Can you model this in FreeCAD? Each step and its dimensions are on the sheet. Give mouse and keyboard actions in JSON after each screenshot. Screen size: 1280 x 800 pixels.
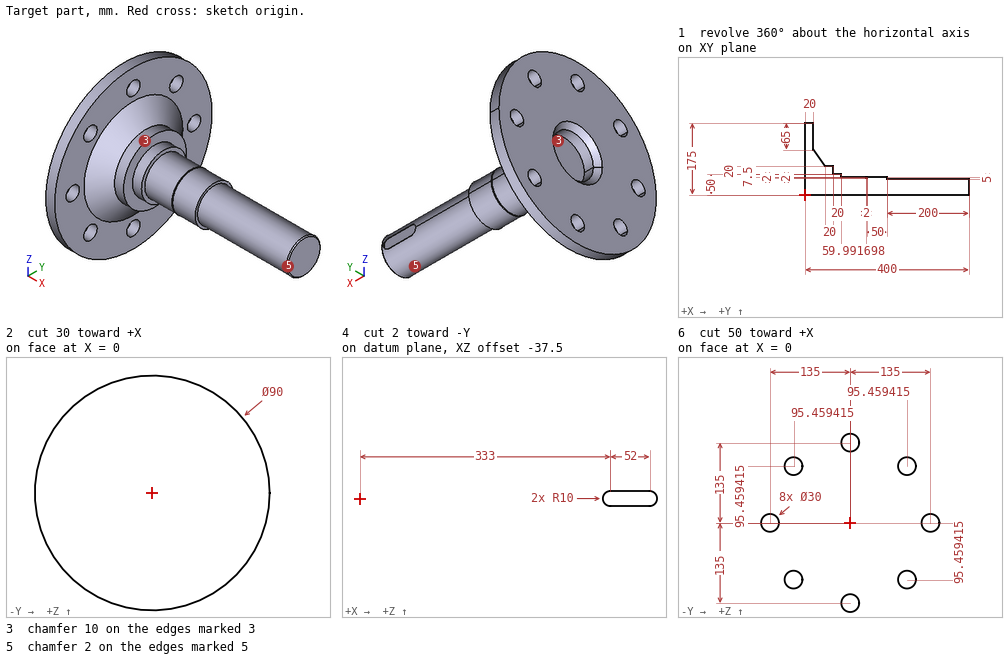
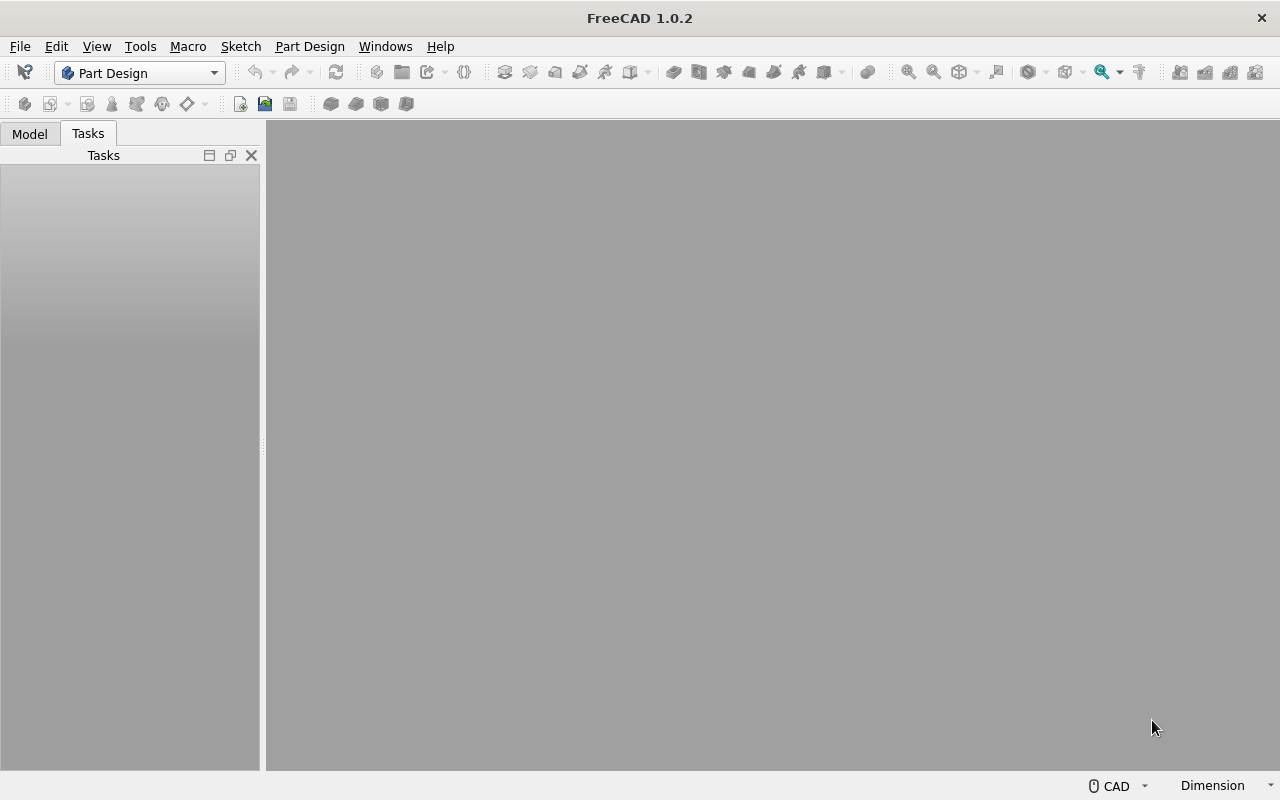
{"action": "left_click", "coordinate": [240, 104]}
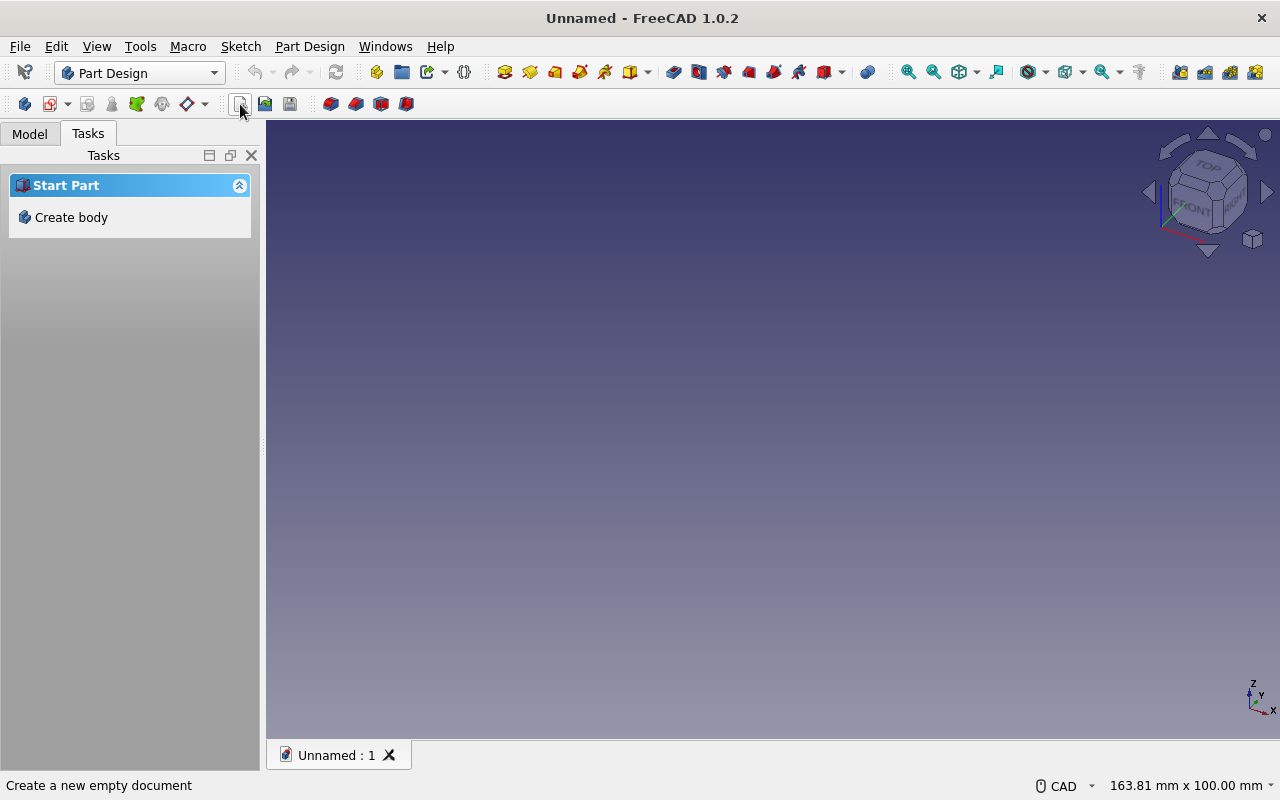
{"action": "left_click", "coordinate": [50, 104]}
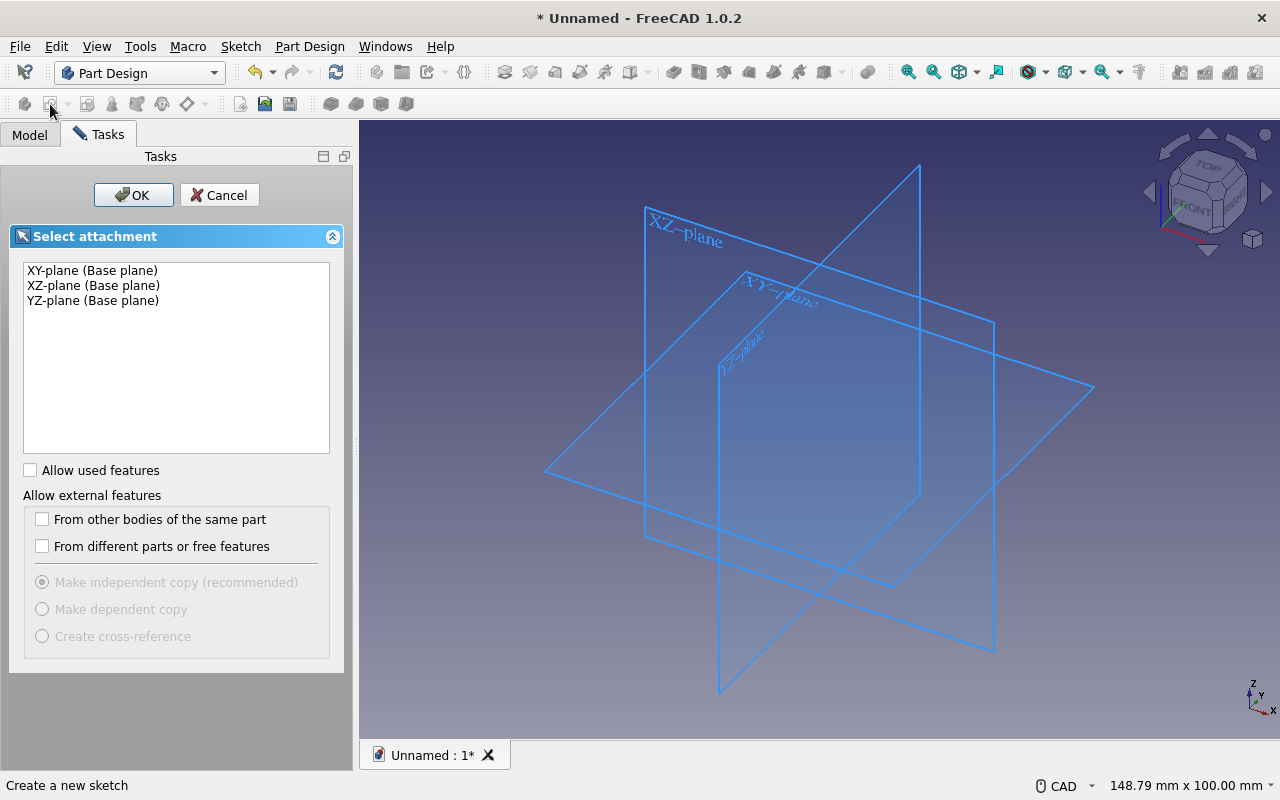
{"action": "left_click", "coordinate": [84, 270]}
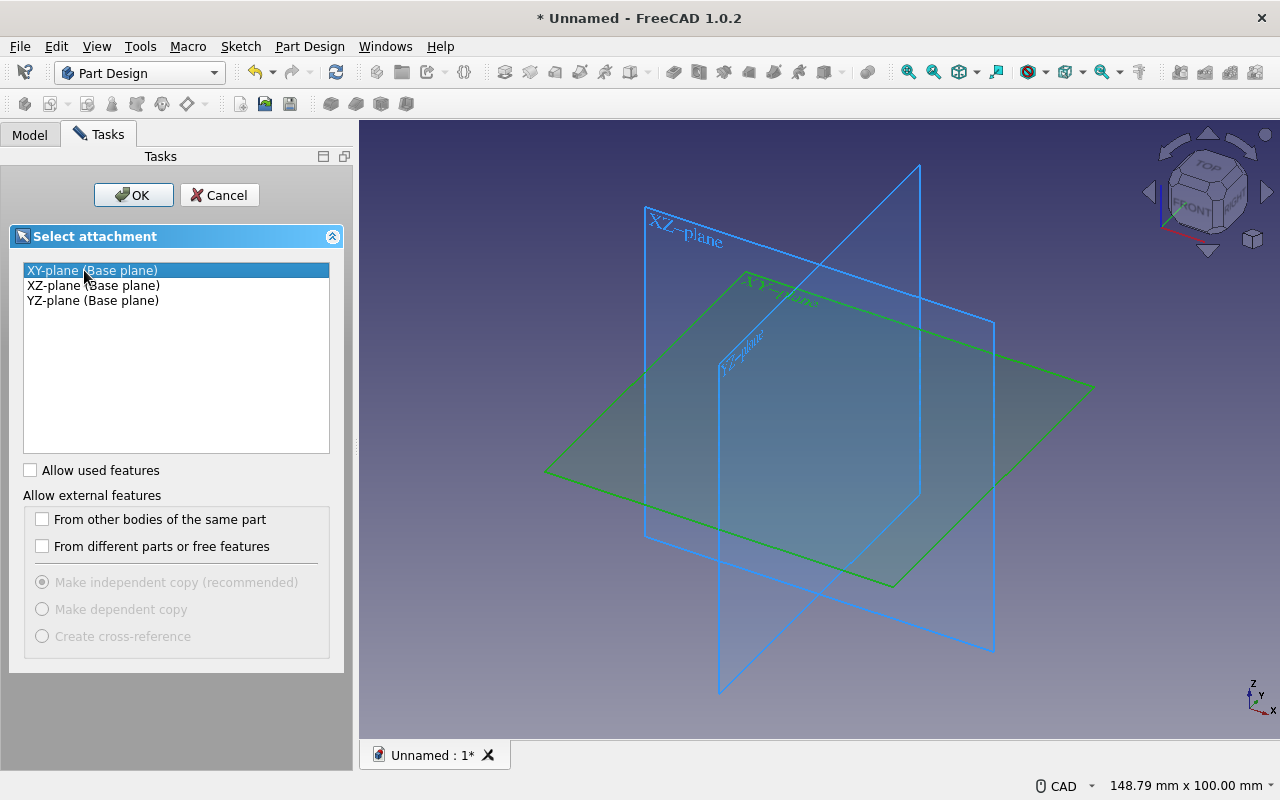
{"action": "left_click", "coordinate": [134, 195]}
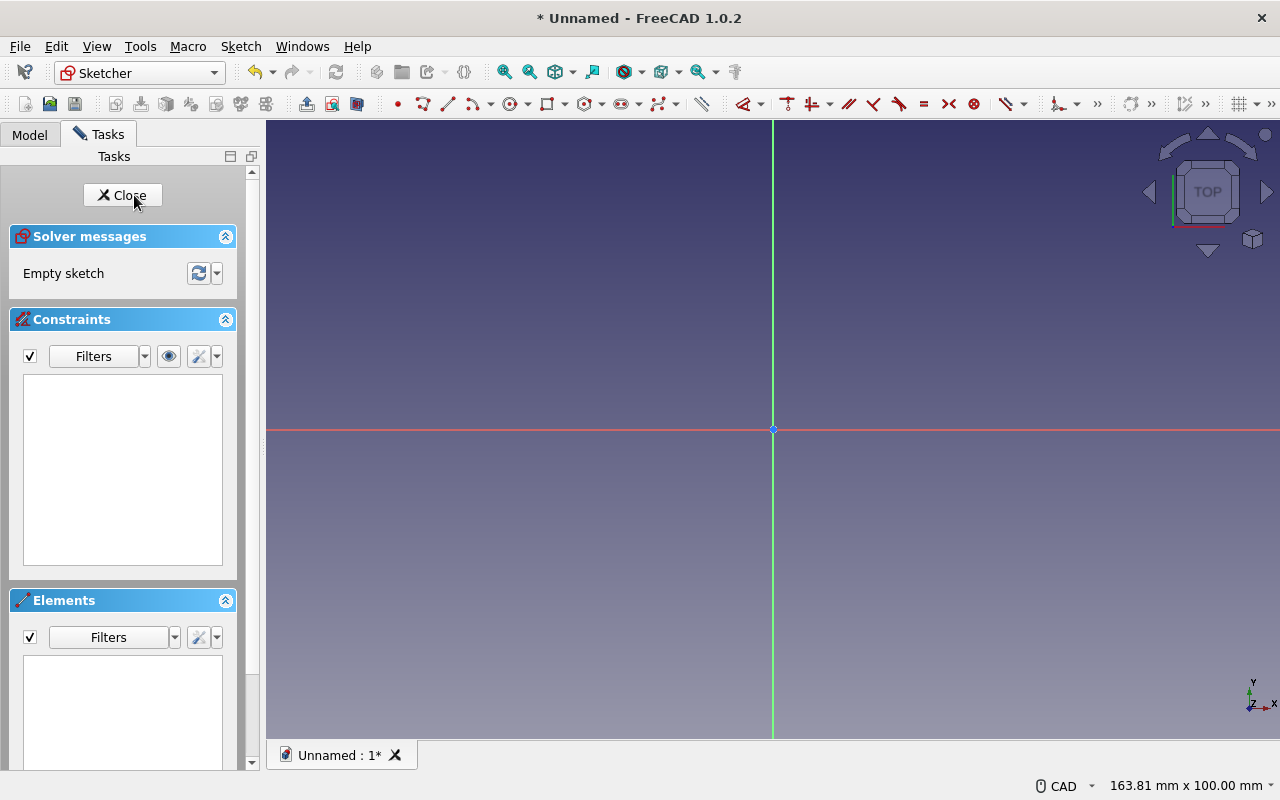
{"action": "scroll", "coordinate": [294, 607], "scroll_direction": "down", "scroll_amount": 7}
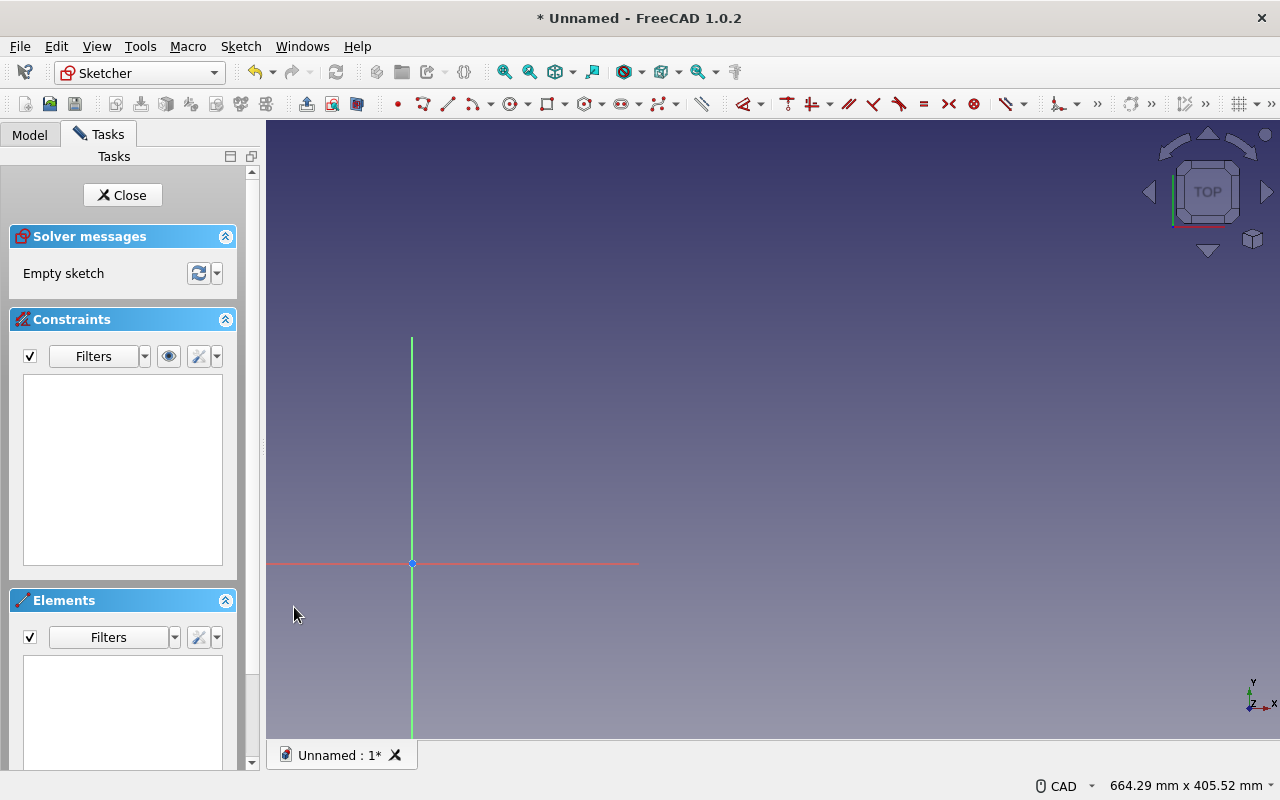
{"action": "left_click", "coordinate": [423, 104]}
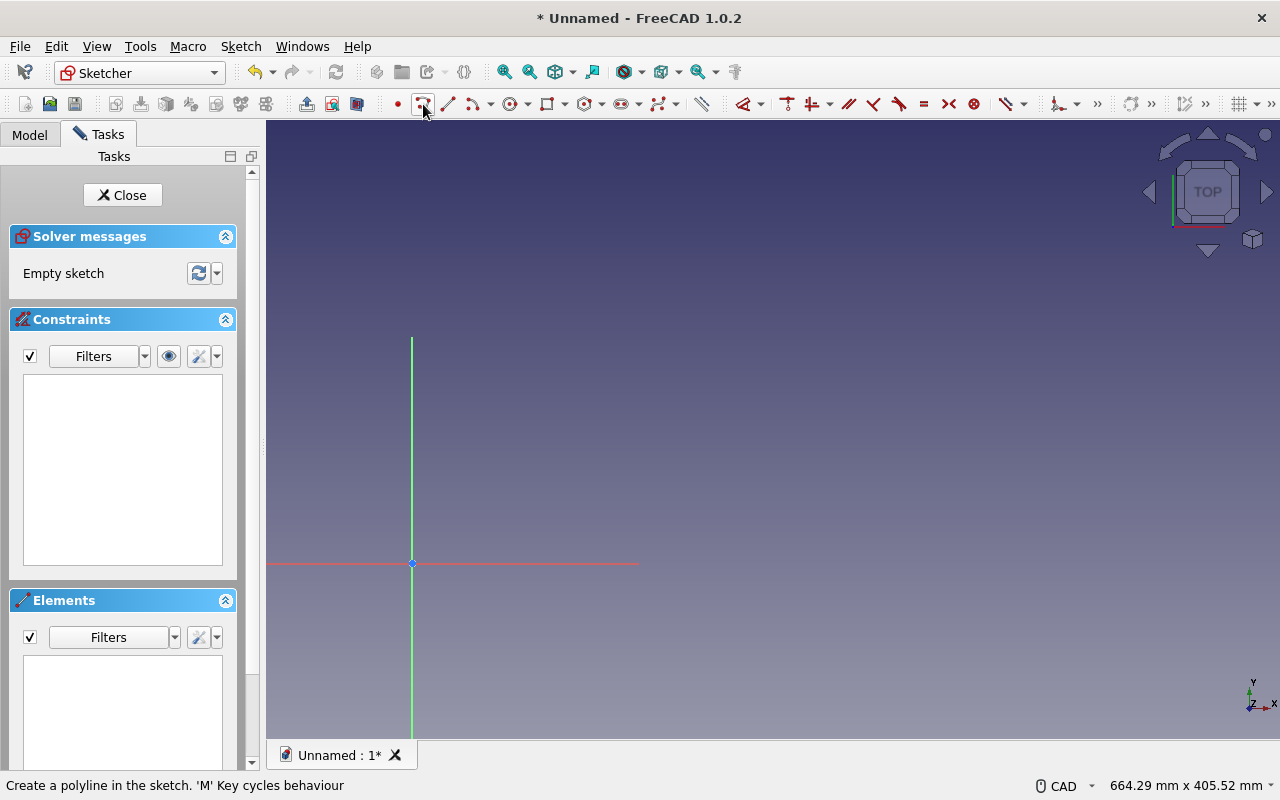
{"action": "left_click", "coordinate": [412, 564]}
{"action": "left_click", "coordinate": [1023, 555]}
{"action": "left_click", "coordinate": [1023, 507]}
{"action": "left_click", "coordinate": [717, 507]}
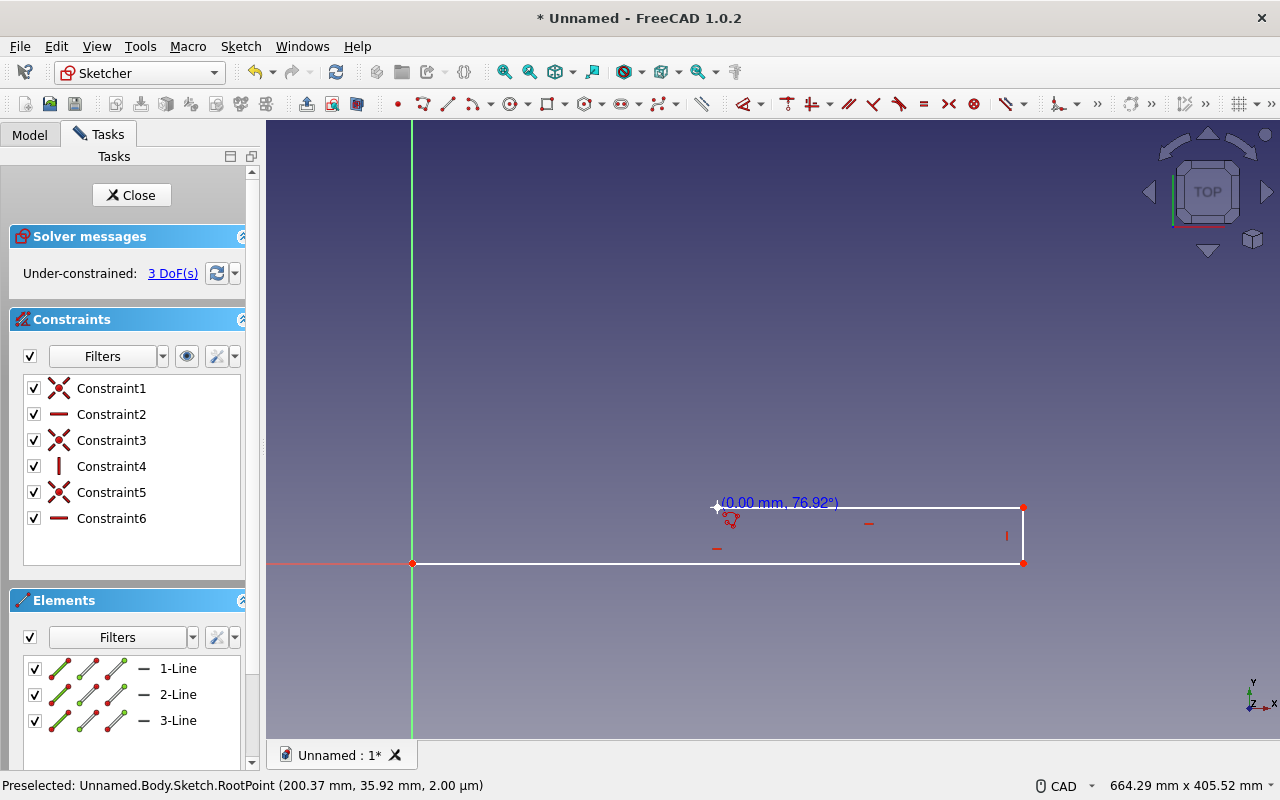
{"action": "scroll", "coordinate": [717, 499], "scroll_direction": "up", "scroll_amount": 4}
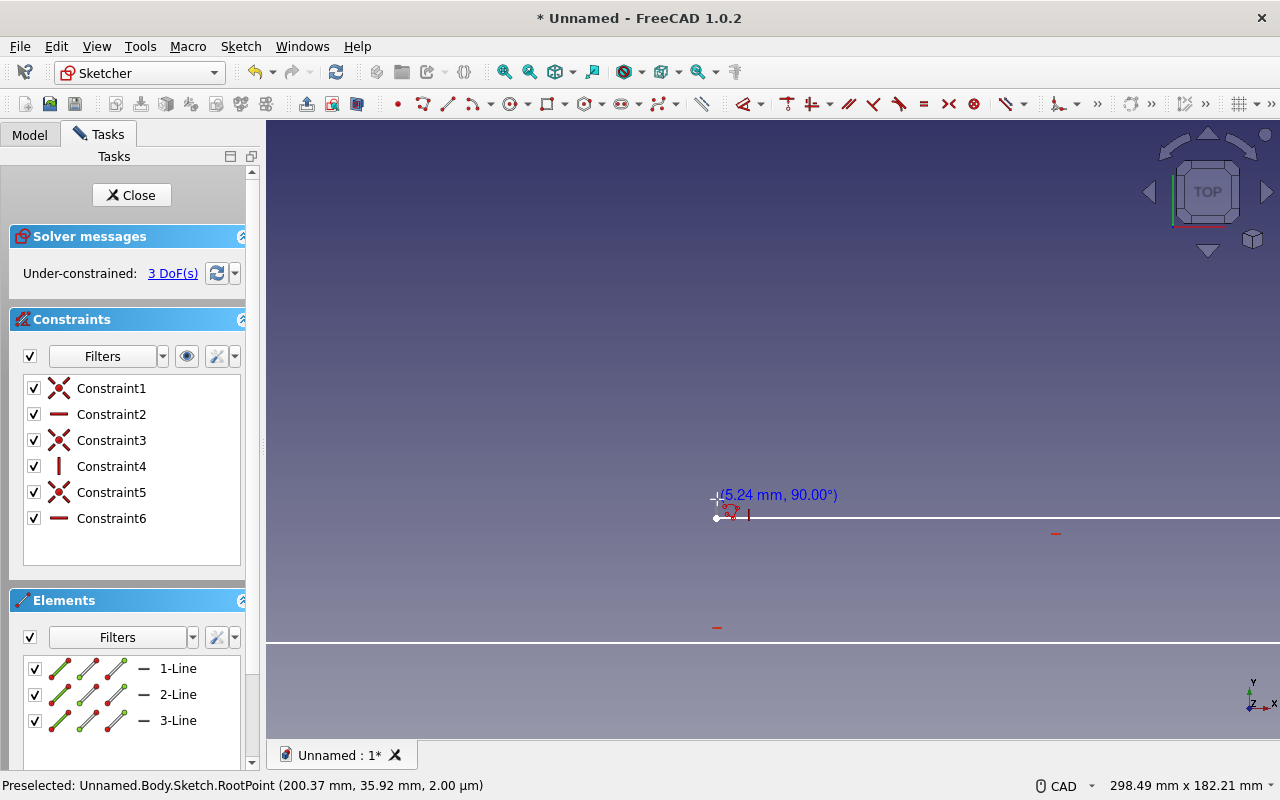
{"action": "left_click", "coordinate": [716, 498]}
{"action": "left_click", "coordinate": [548, 498]}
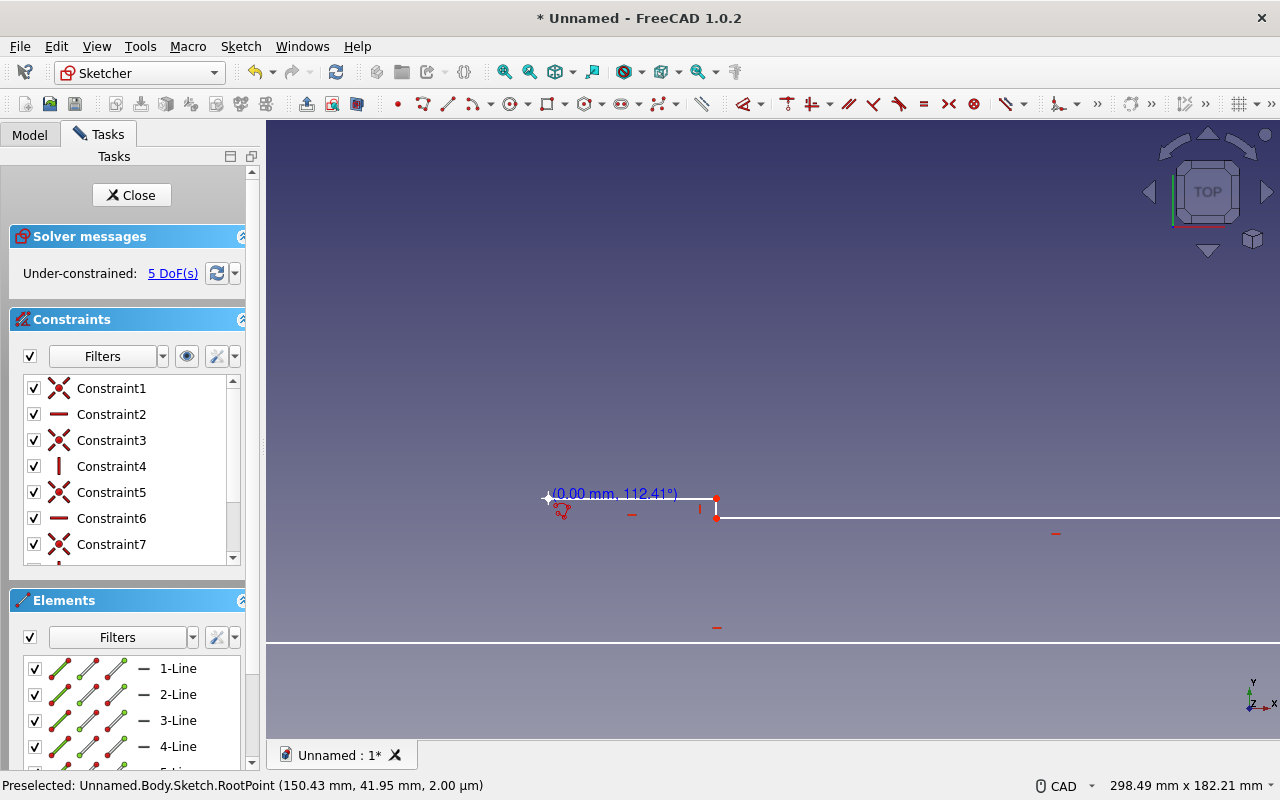
{"action": "scroll", "coordinate": [548, 505], "scroll_direction": "up", "scroll_amount": 5}